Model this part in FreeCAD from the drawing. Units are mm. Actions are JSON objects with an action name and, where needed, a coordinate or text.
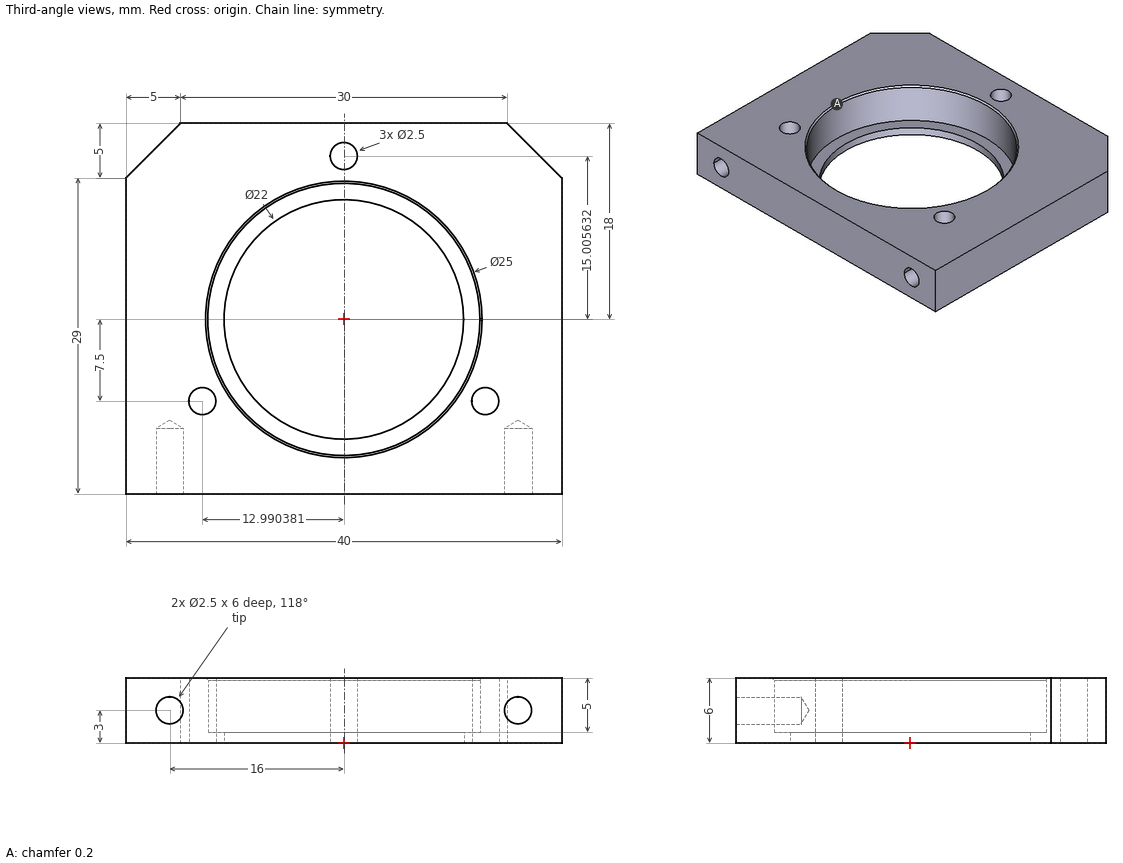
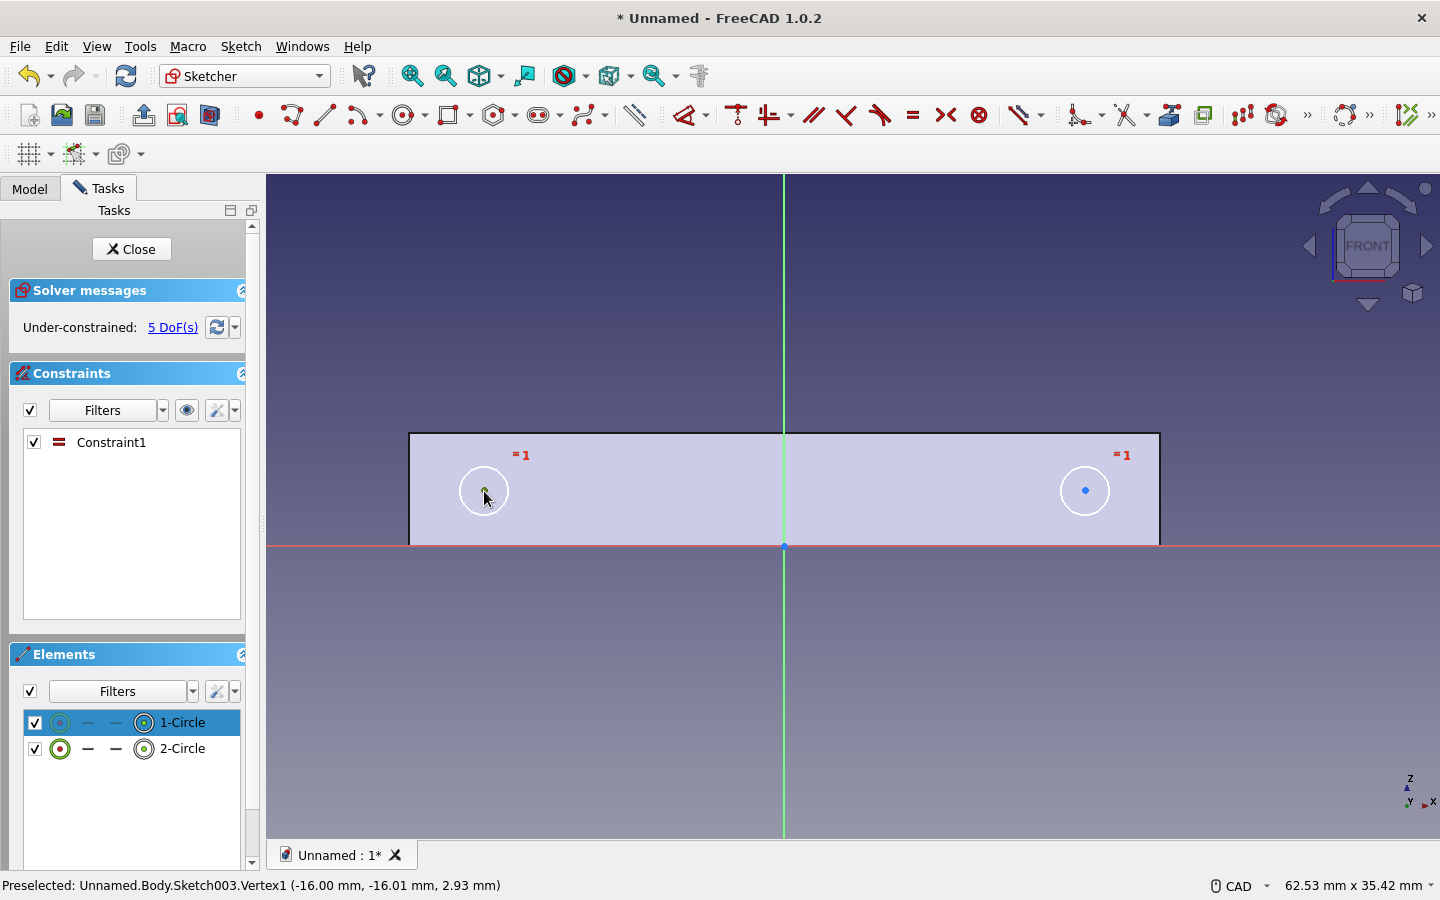
{"action": "left_click", "coordinate": [1085, 491]}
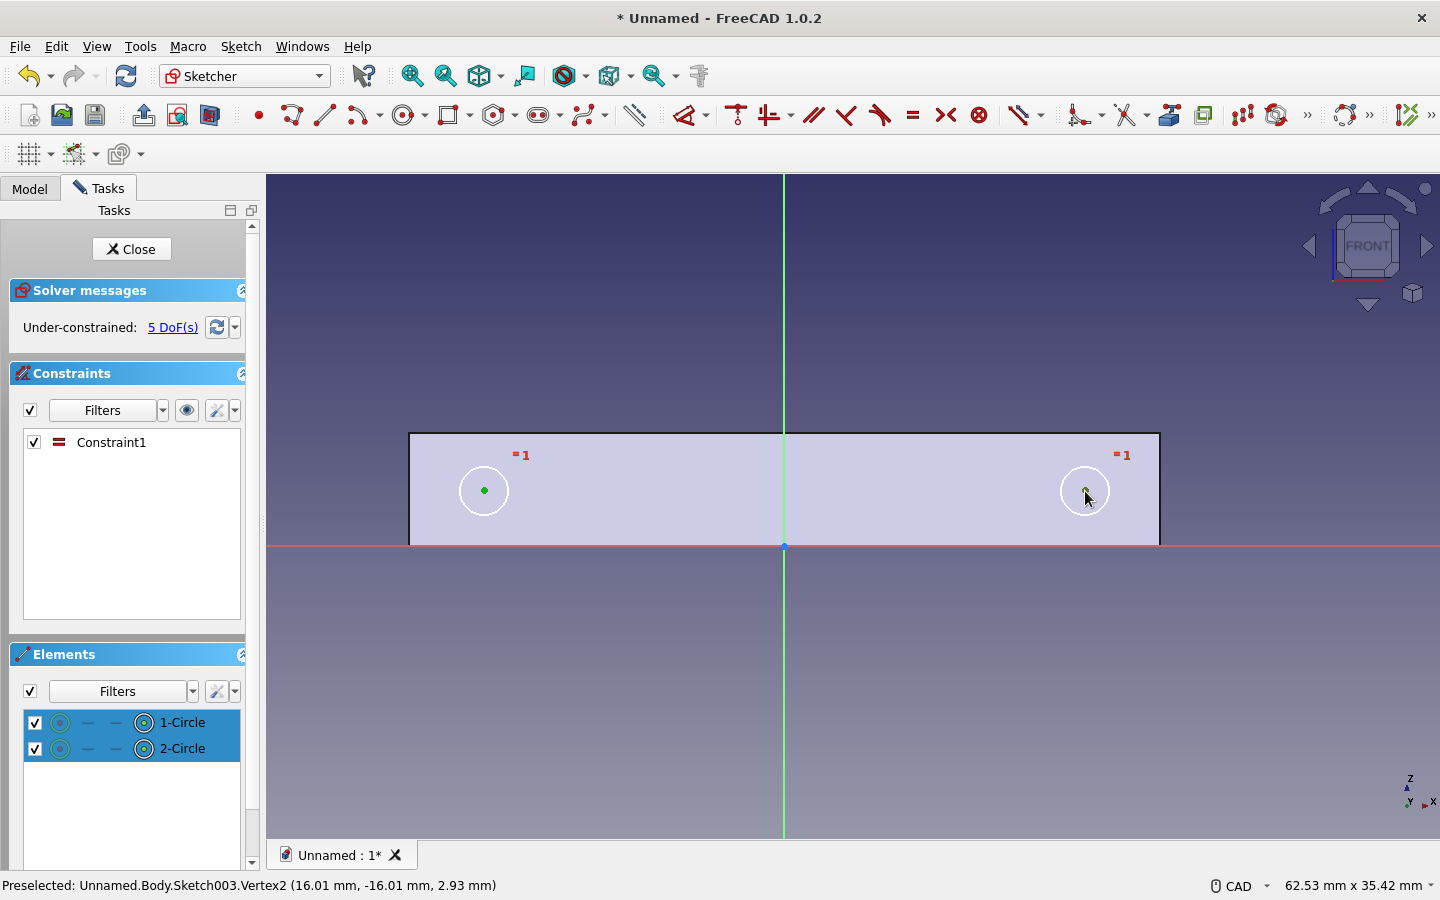
{"action": "left_click", "coordinate": [784, 768]}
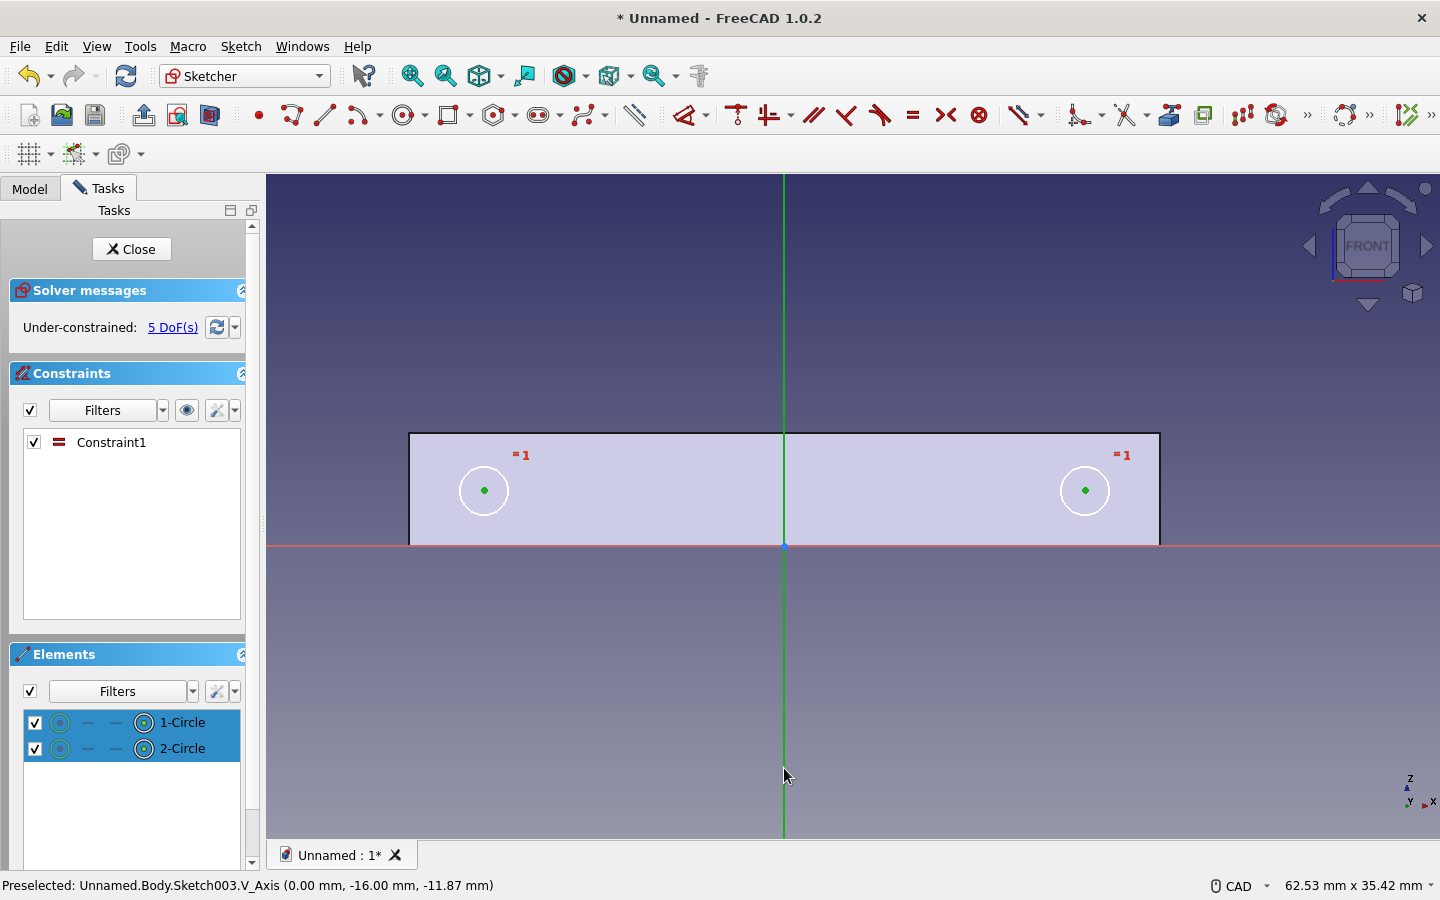
{"action": "left_click", "coordinate": [946, 116]}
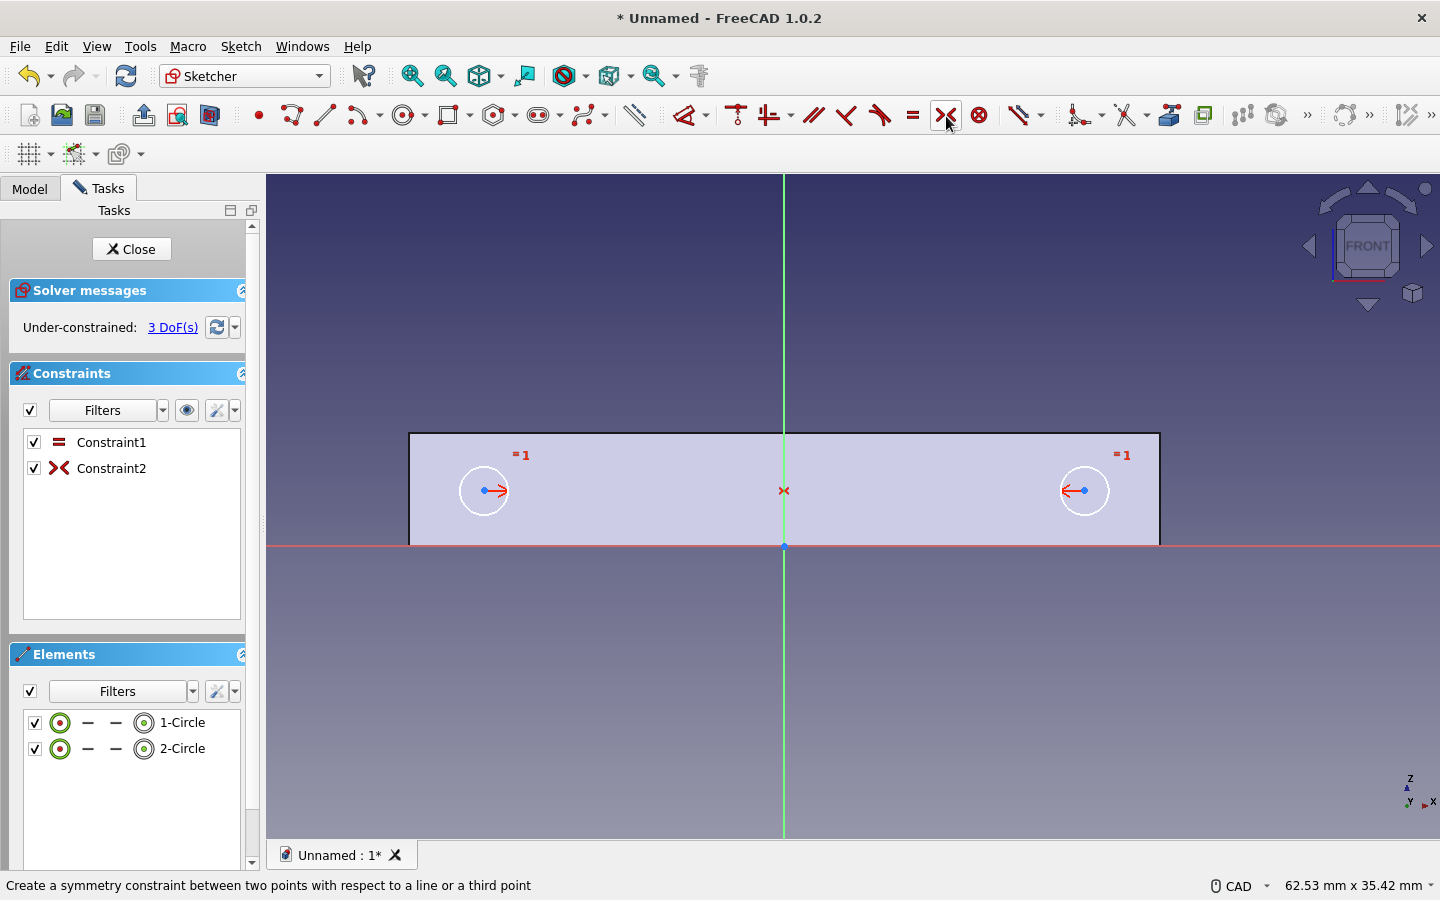
{"action": "left_click", "coordinate": [684, 116]}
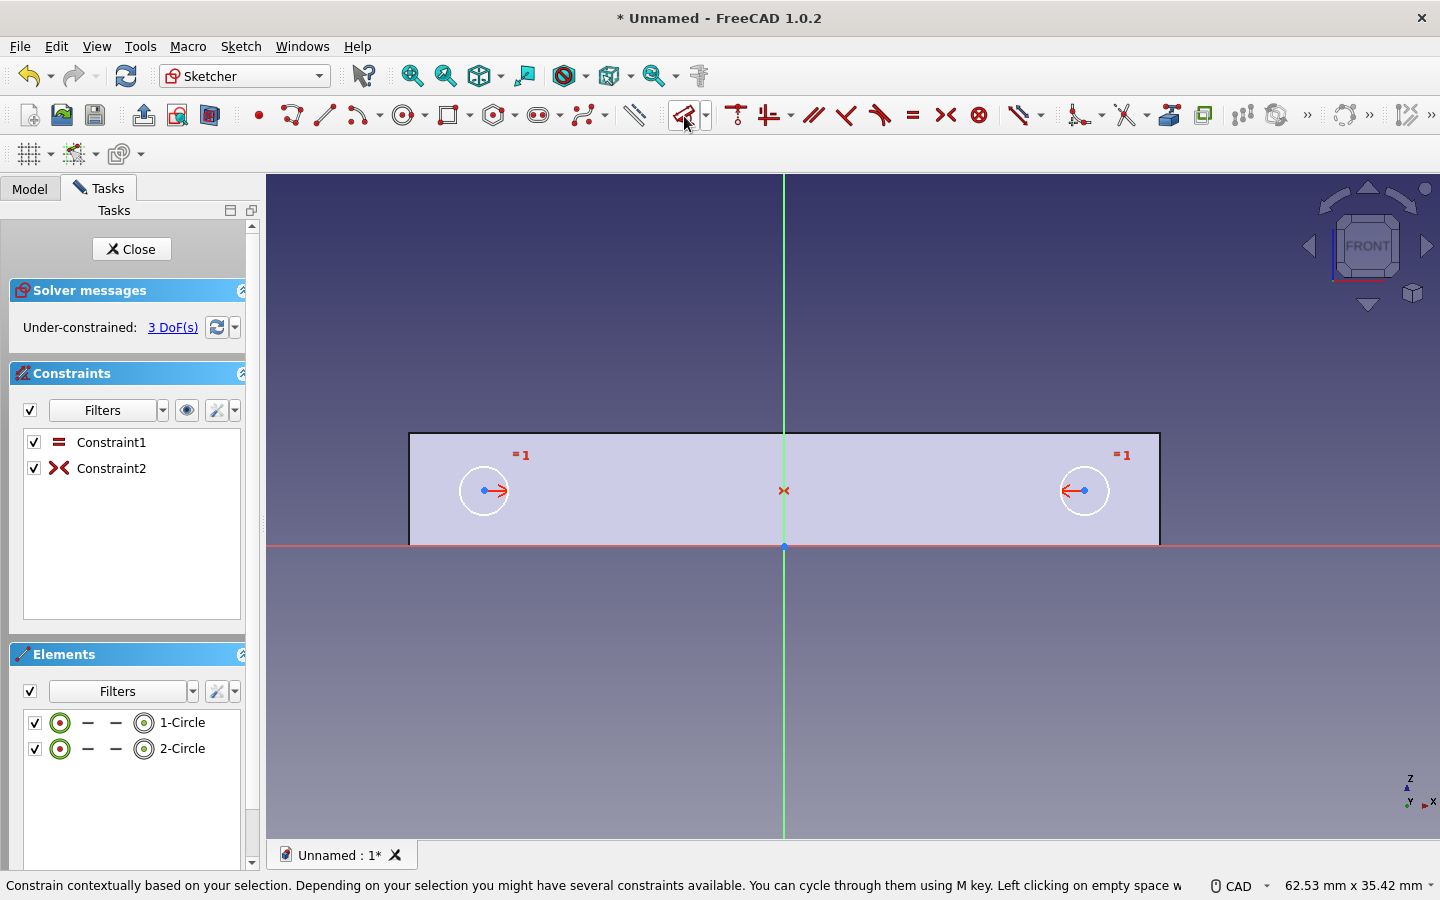
{"action": "left_click", "coordinate": [501, 474]}
{"action": "left_click", "coordinate": [524, 451]}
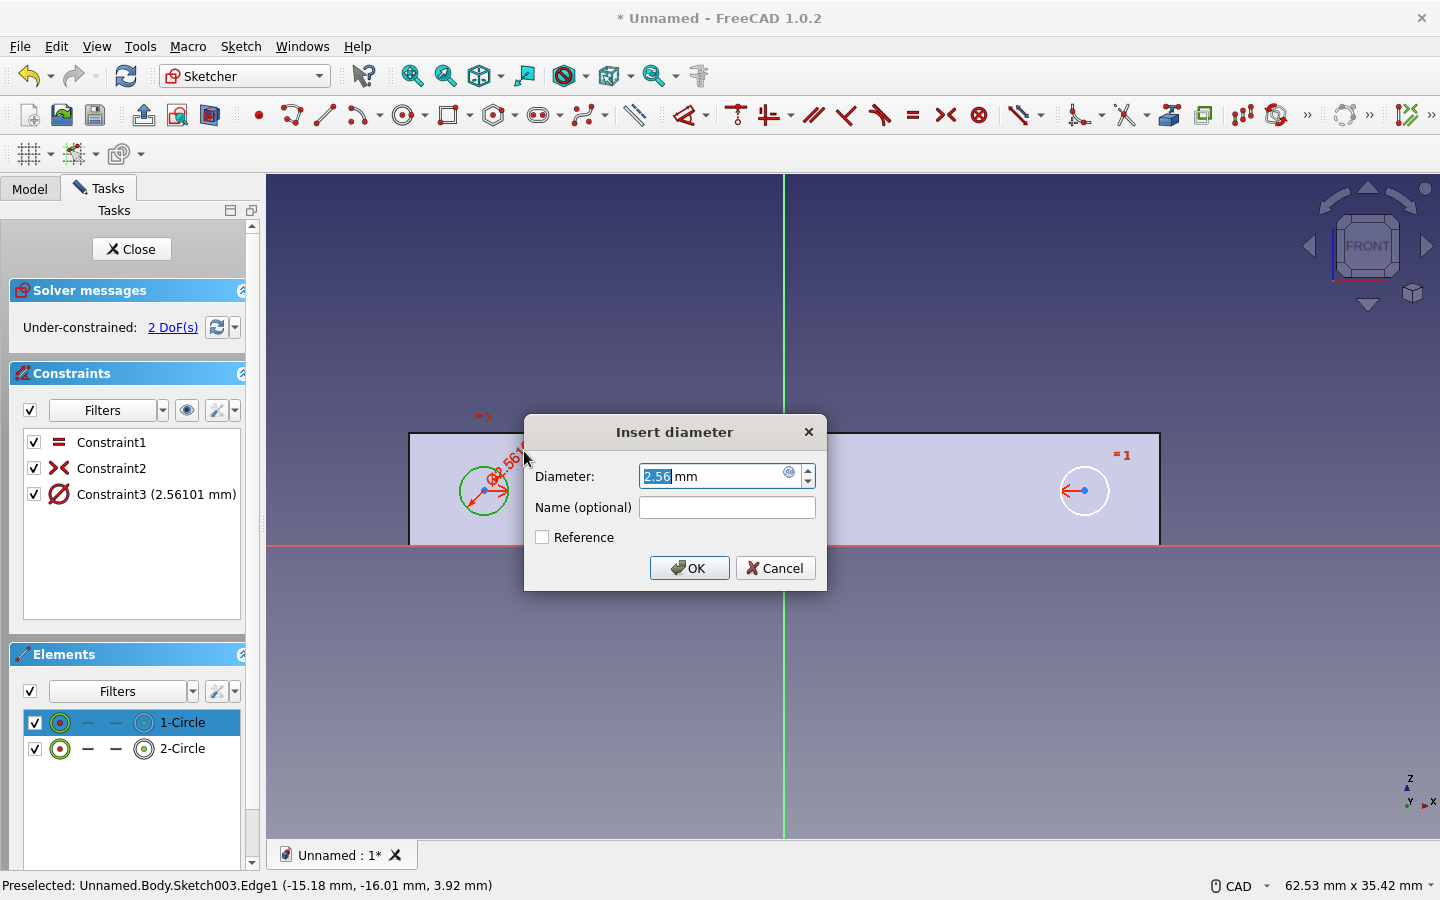
{"action": "type", "text": "2.5"}
{"action": "key", "text": "Return"}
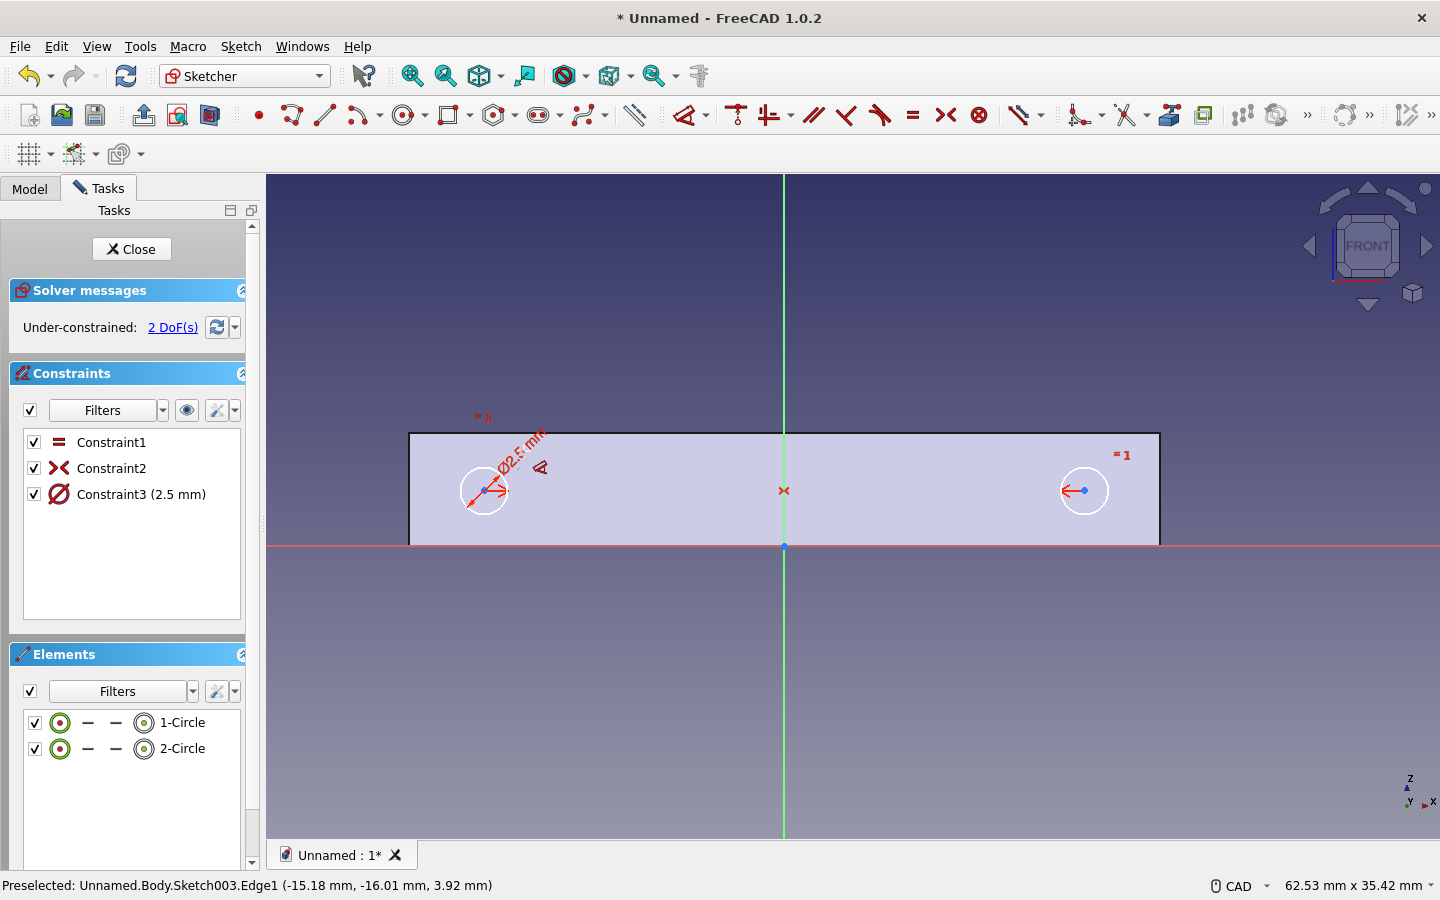
{"action": "left_click", "coordinate": [484, 491]}
{"action": "left_click", "coordinate": [450, 519]}